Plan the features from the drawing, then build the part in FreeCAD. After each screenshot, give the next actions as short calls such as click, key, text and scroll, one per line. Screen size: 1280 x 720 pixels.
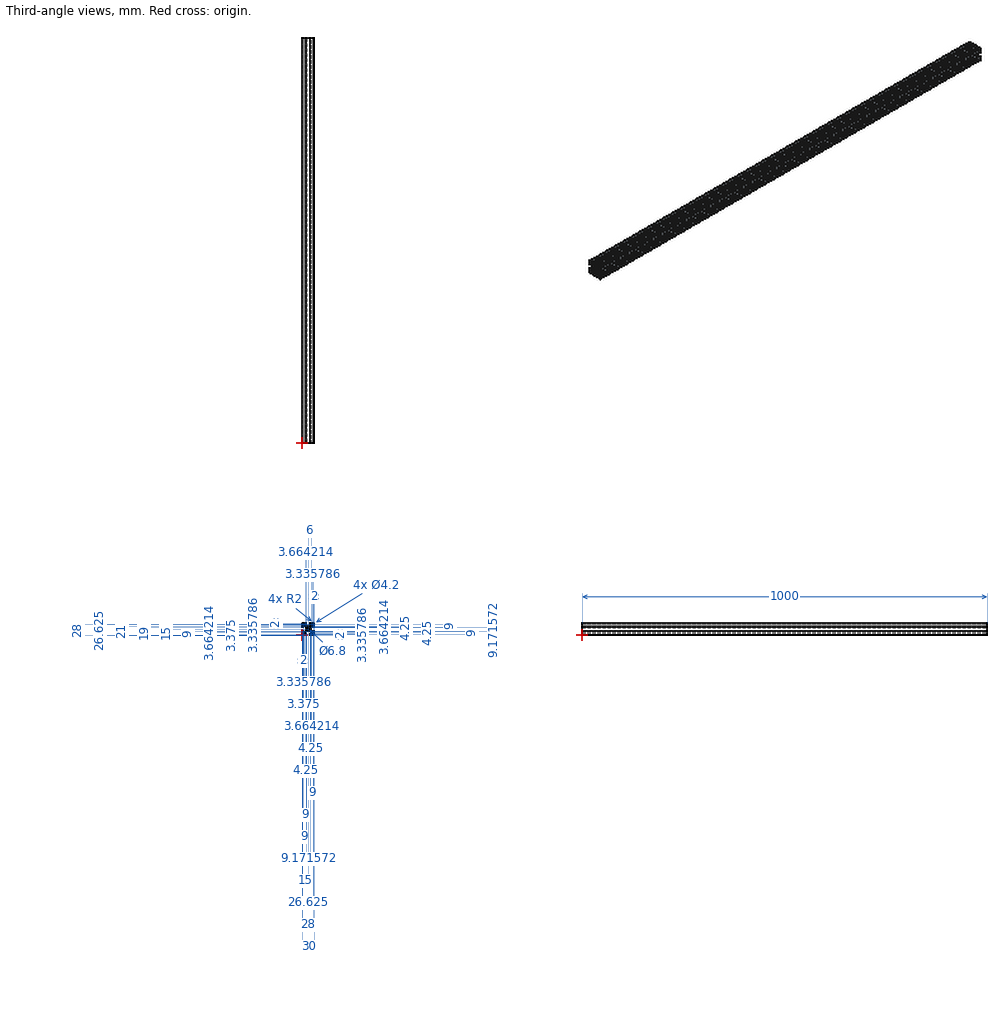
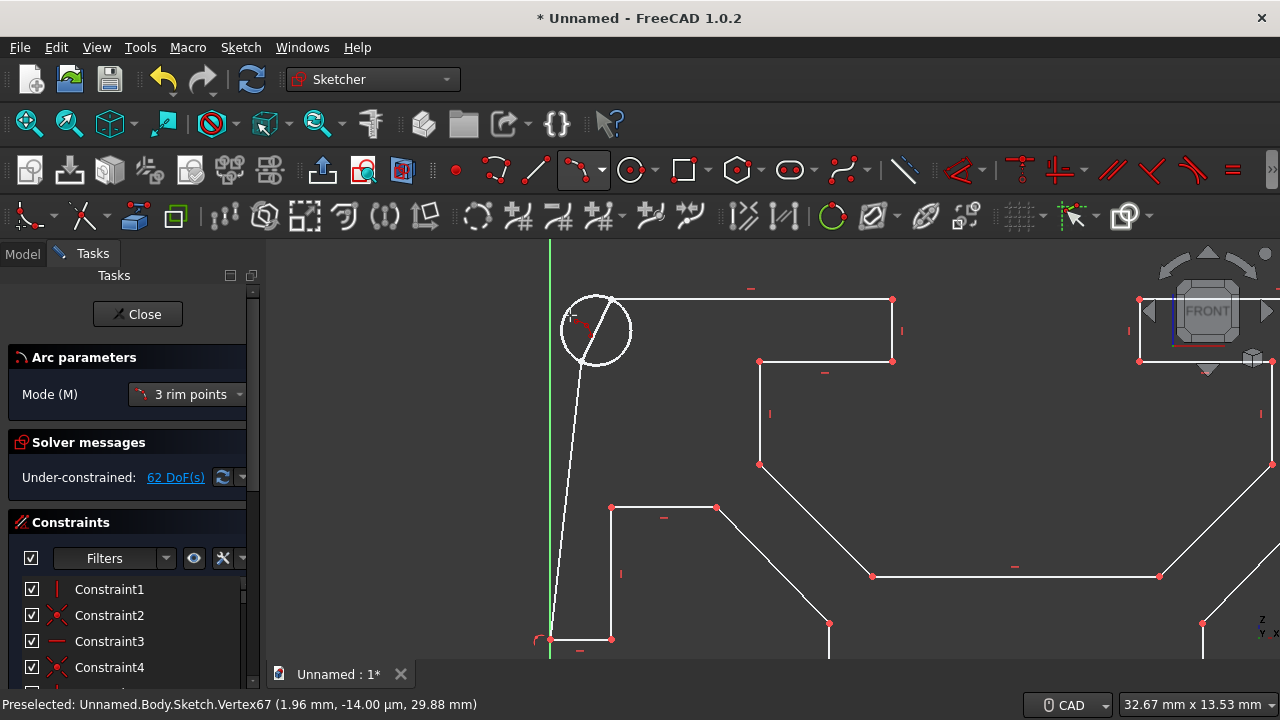
click(569, 314)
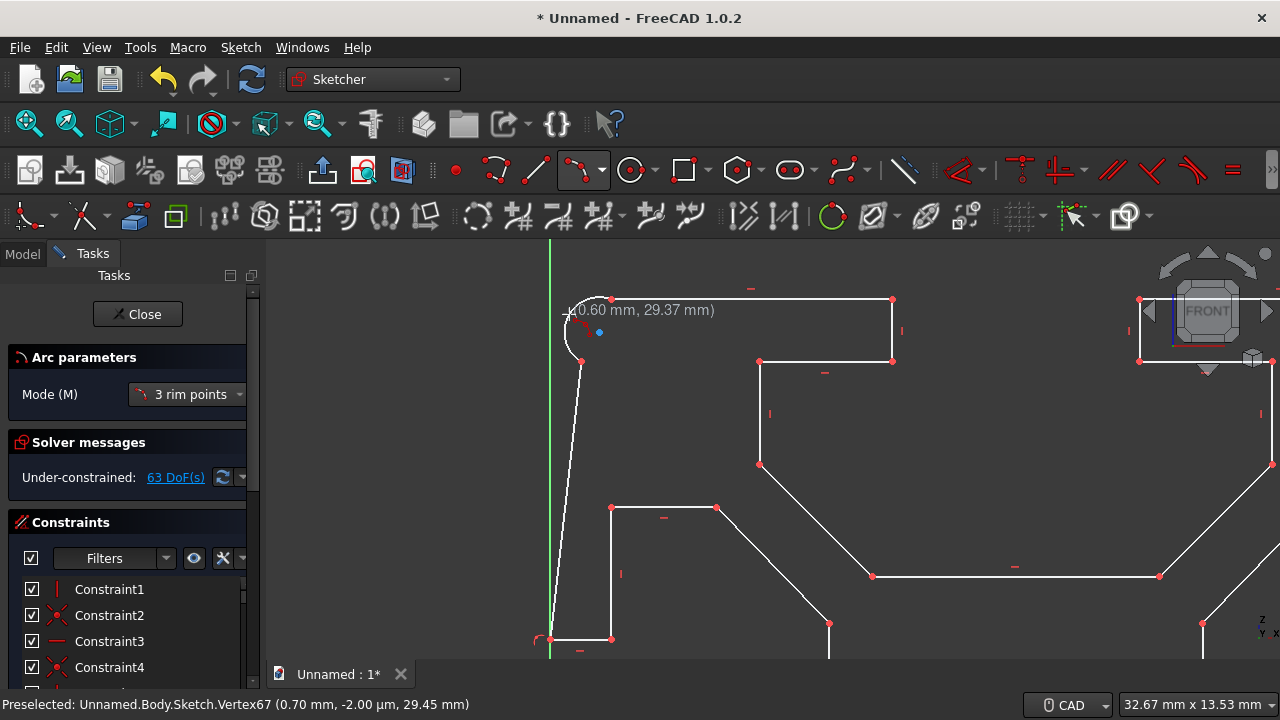
scroll(570, 314, down, 6)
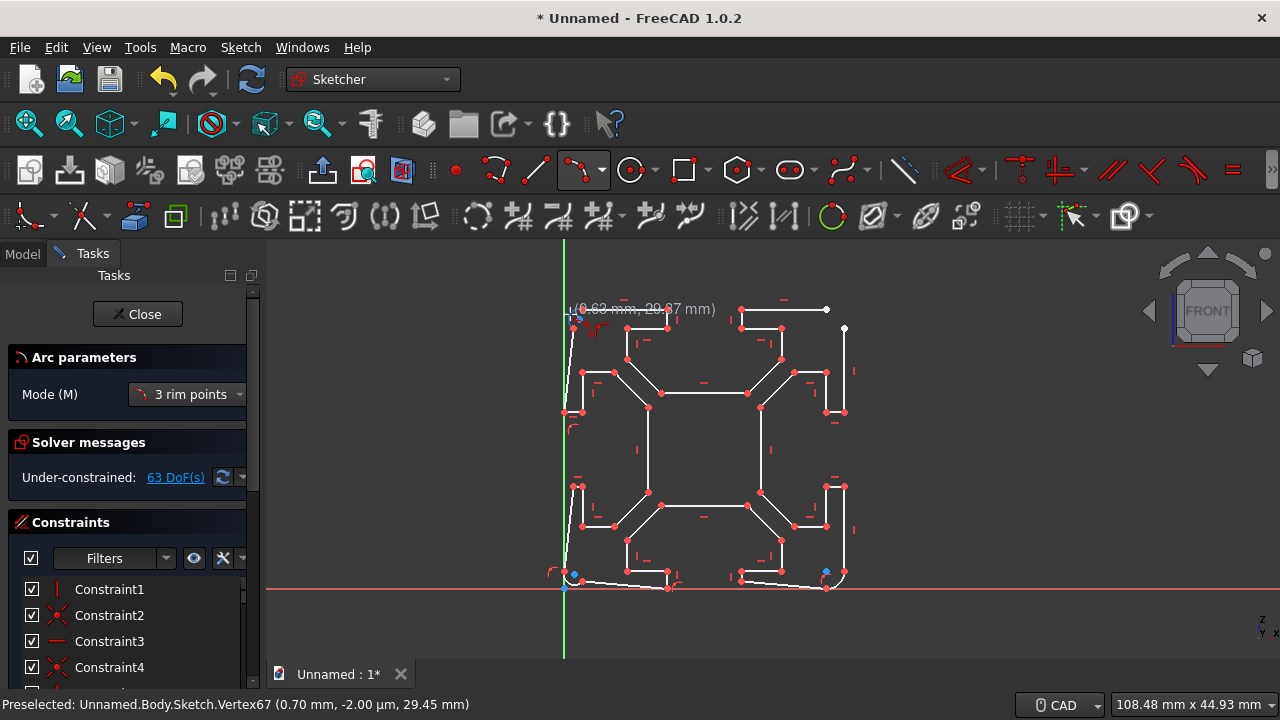
click(826, 310)
click(844, 329)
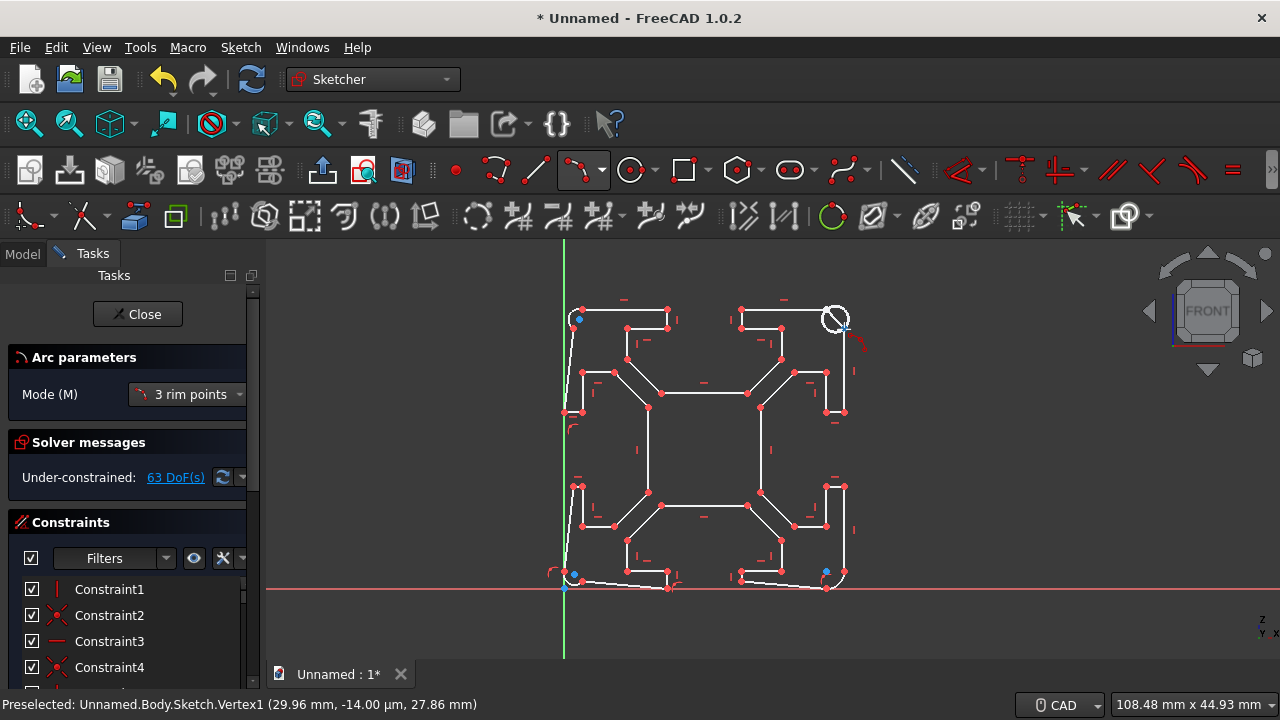
scroll(839, 314, up, 6)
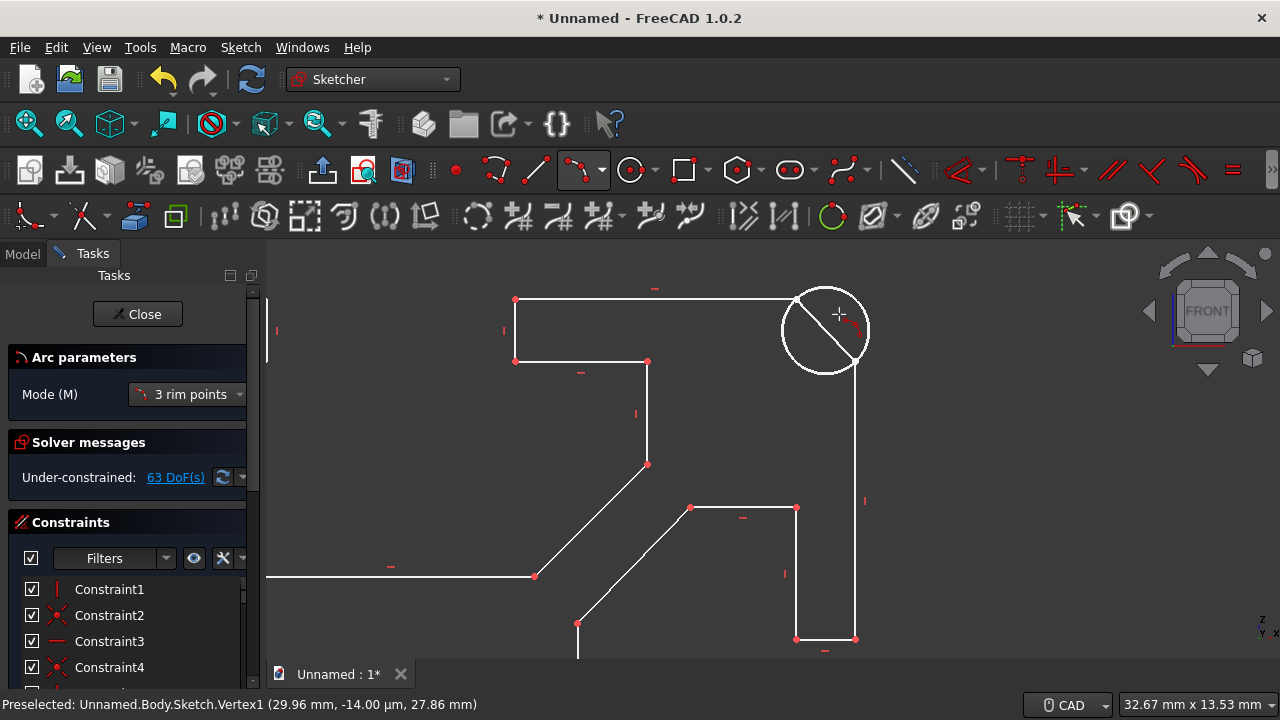
click(839, 314)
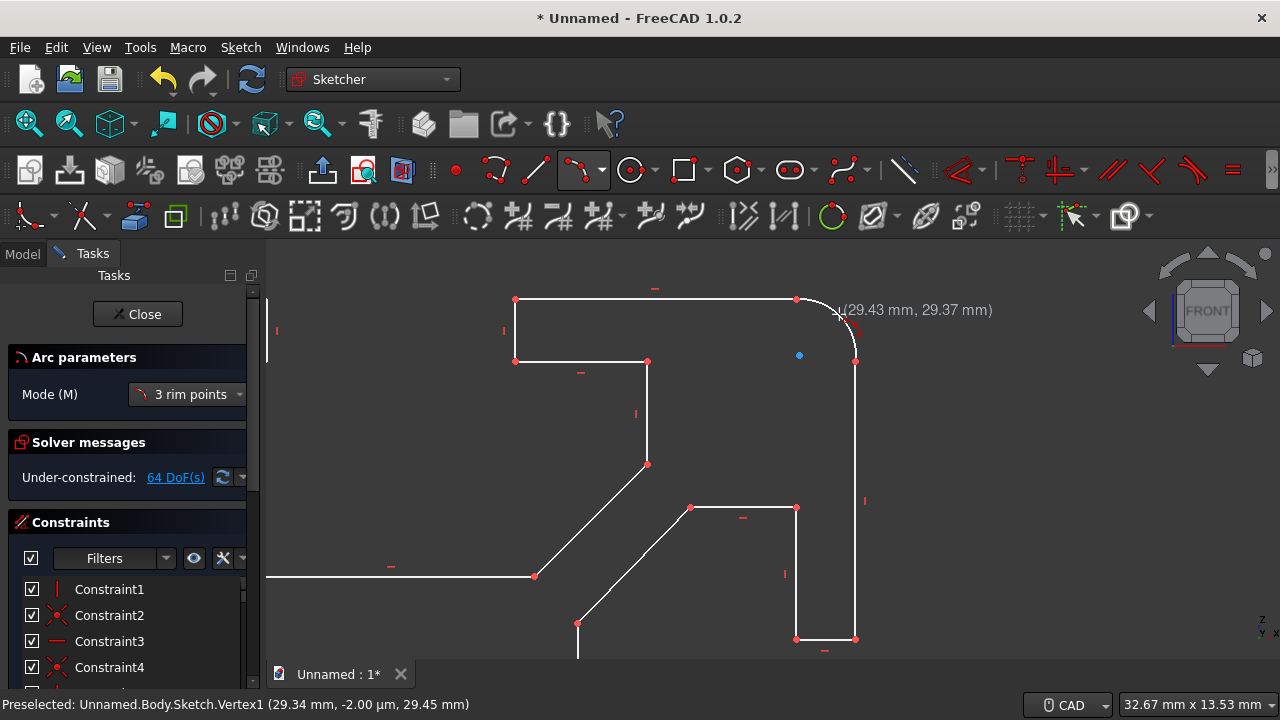
click(632, 170)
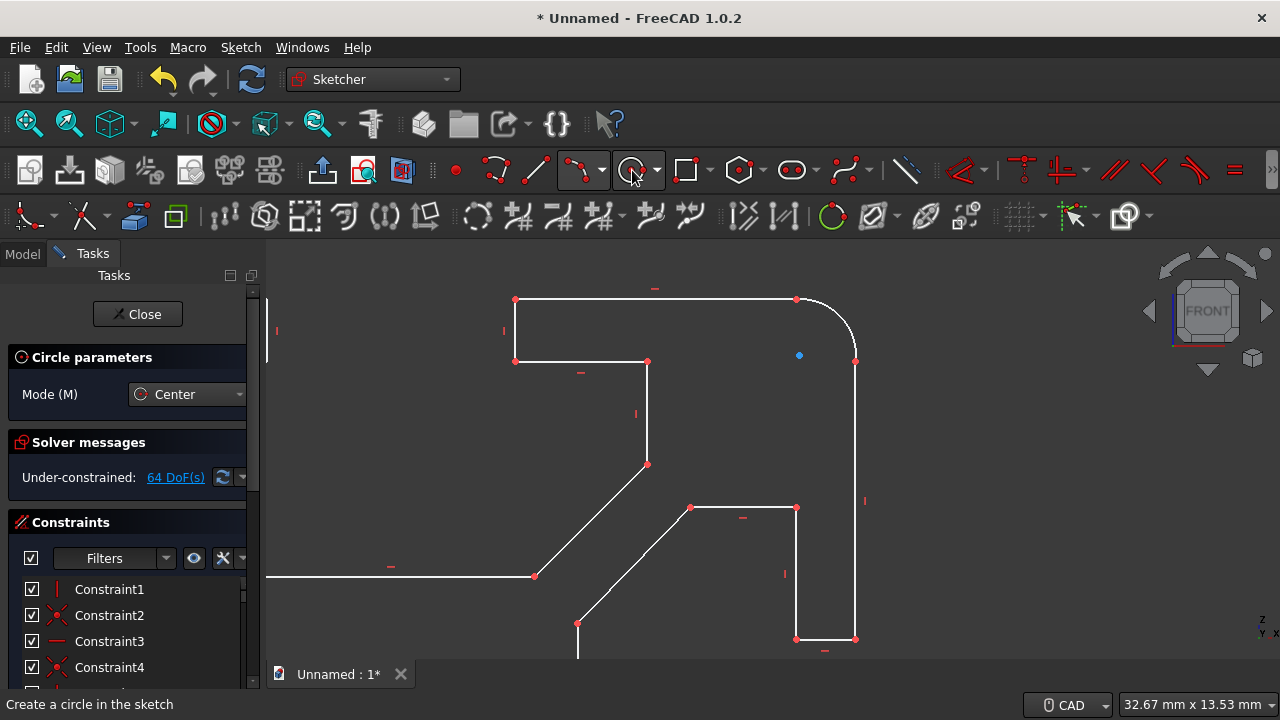
click(752, 400)
move(706, 354)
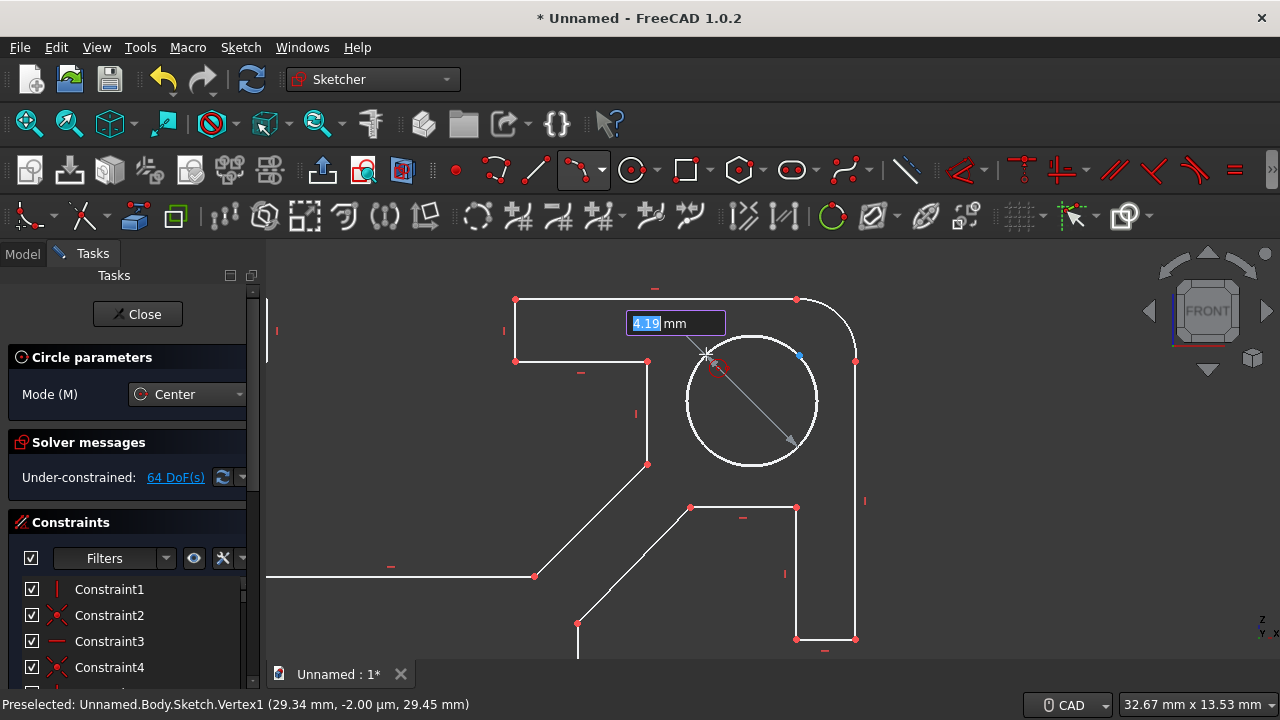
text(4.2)
key(Return)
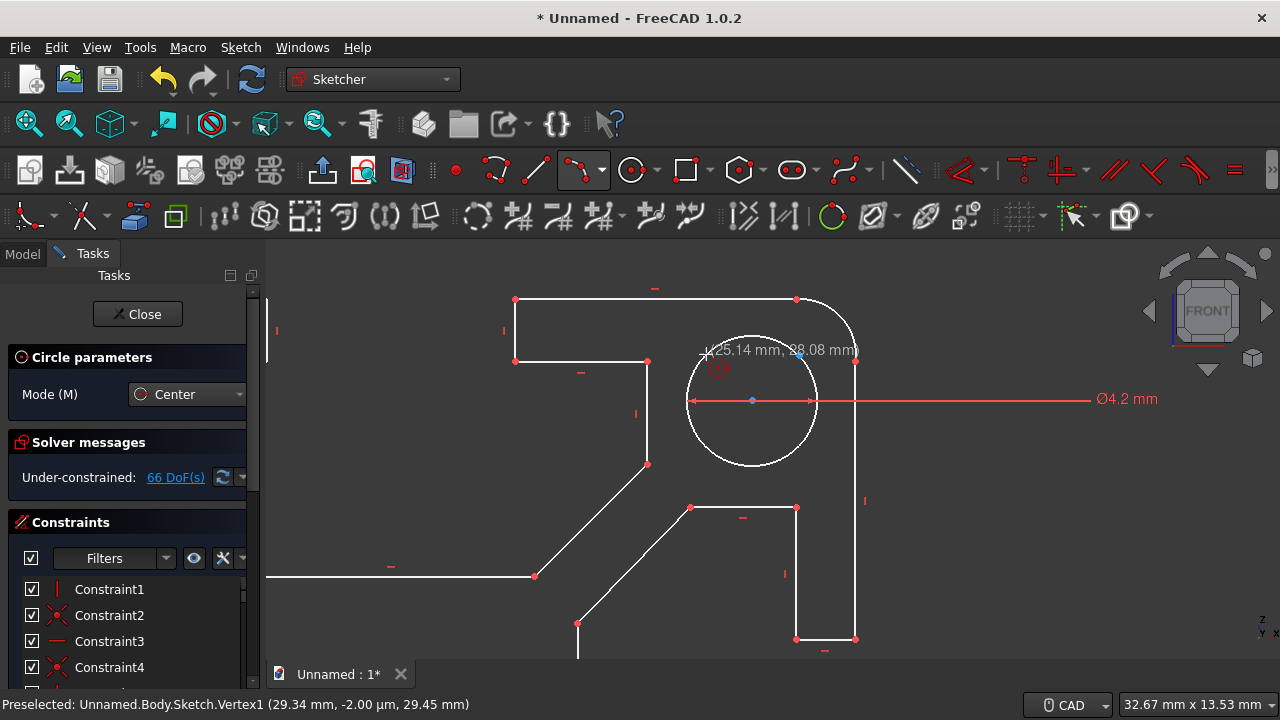
scroll(840, 314, down, 6)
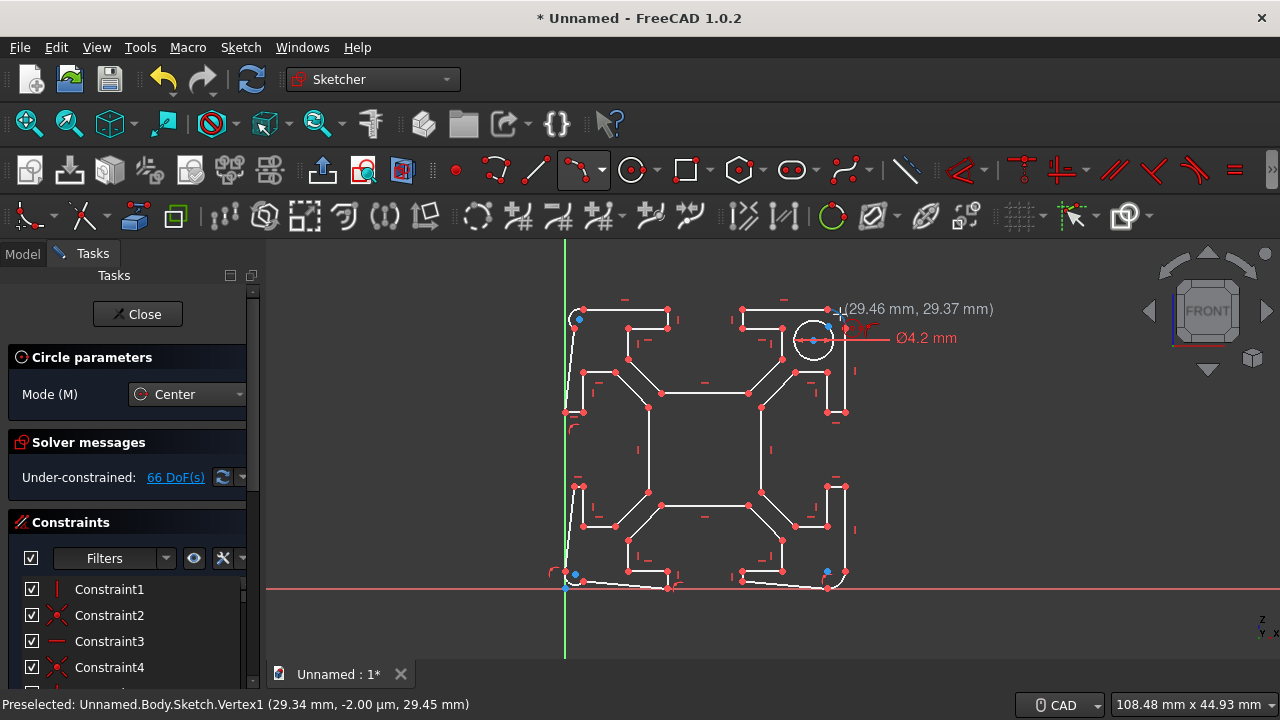
click(597, 340)
move(610, 326)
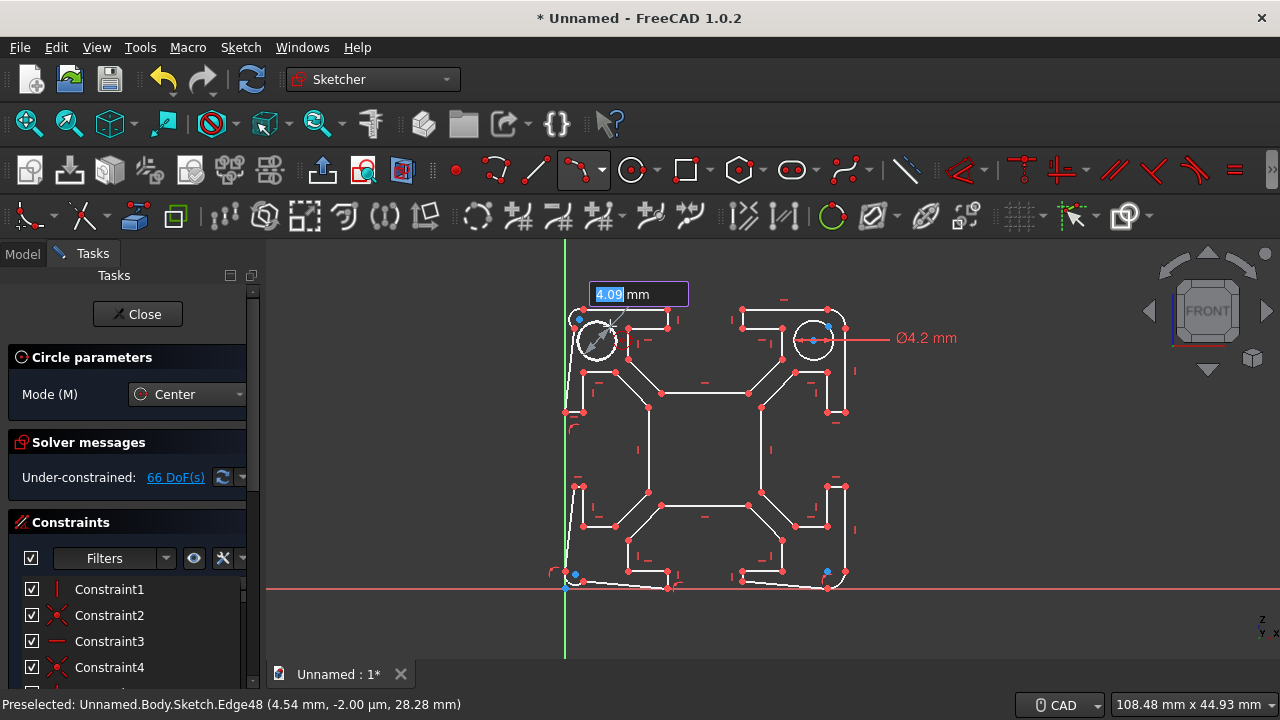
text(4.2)
key(Return)